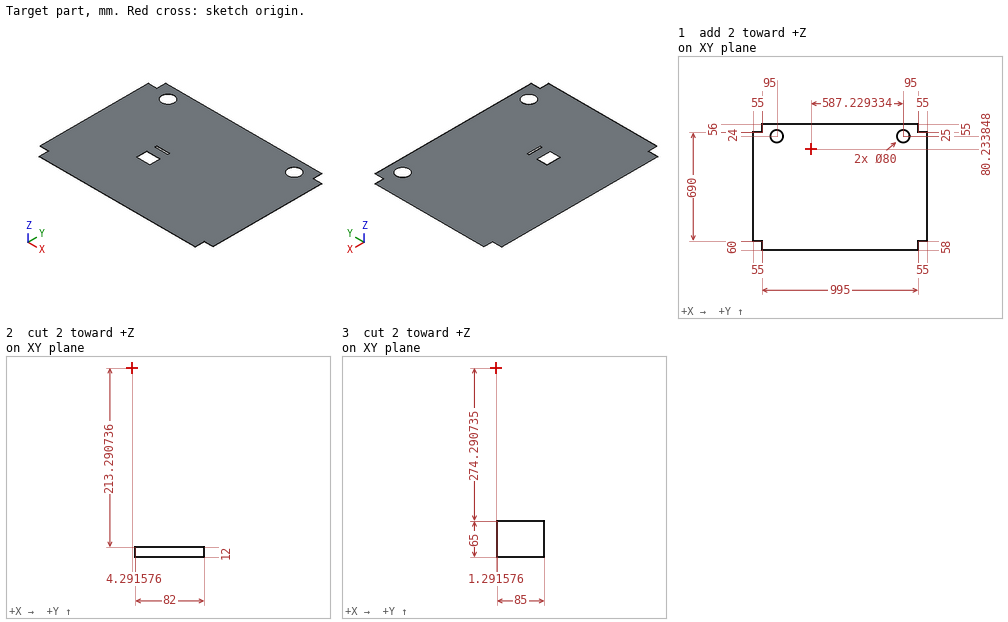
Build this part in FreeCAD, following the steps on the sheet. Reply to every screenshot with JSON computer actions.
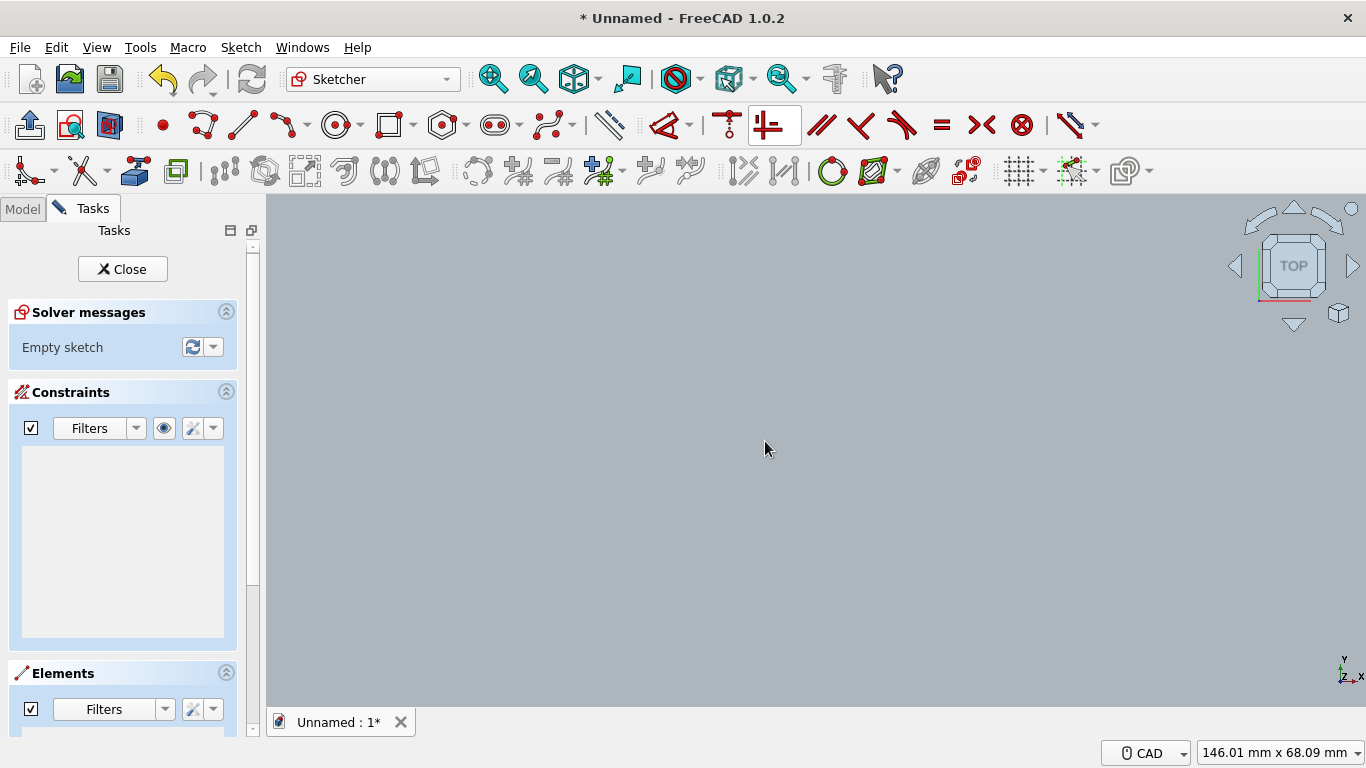
{"action": "left_click", "coordinate": [390, 126]}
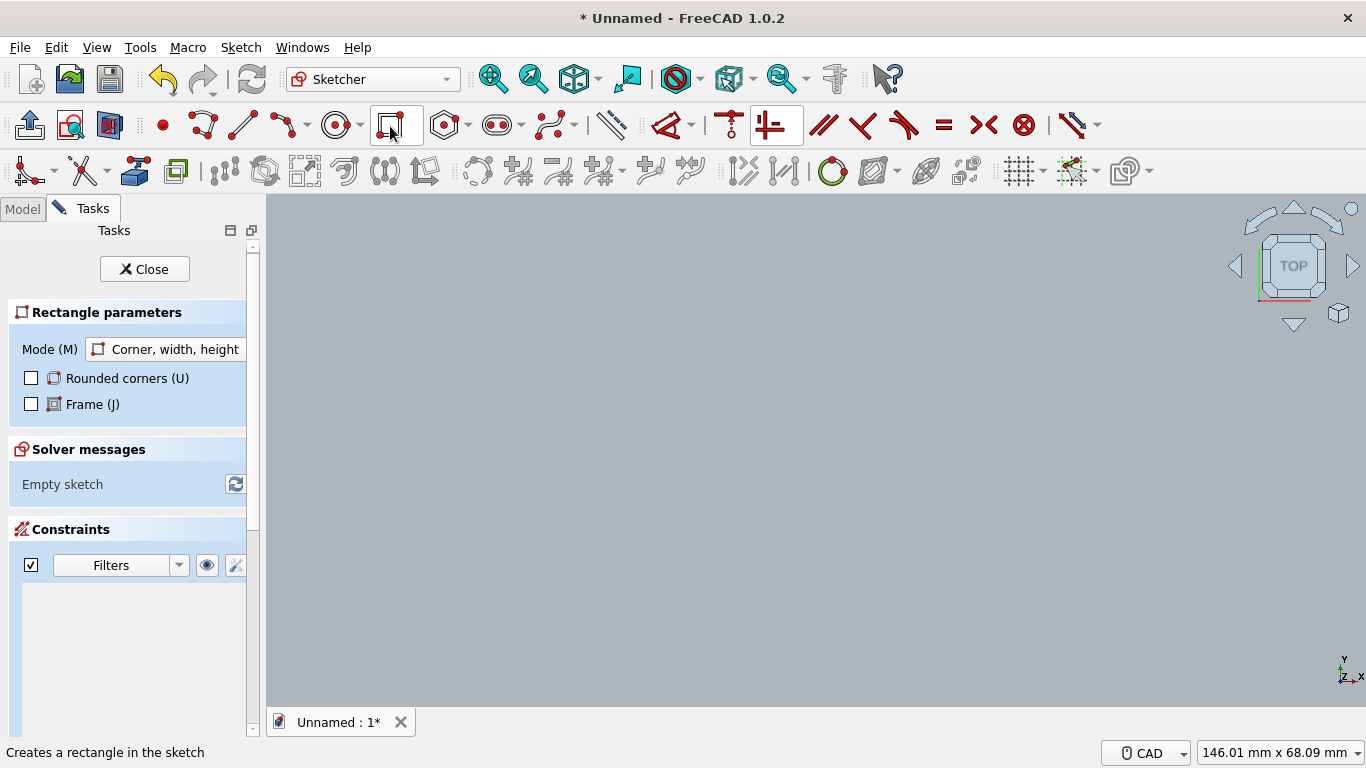
{"action": "left_click", "coordinate": [421, 401]}
{"action": "mouse_move", "coordinate": [1039, 491]}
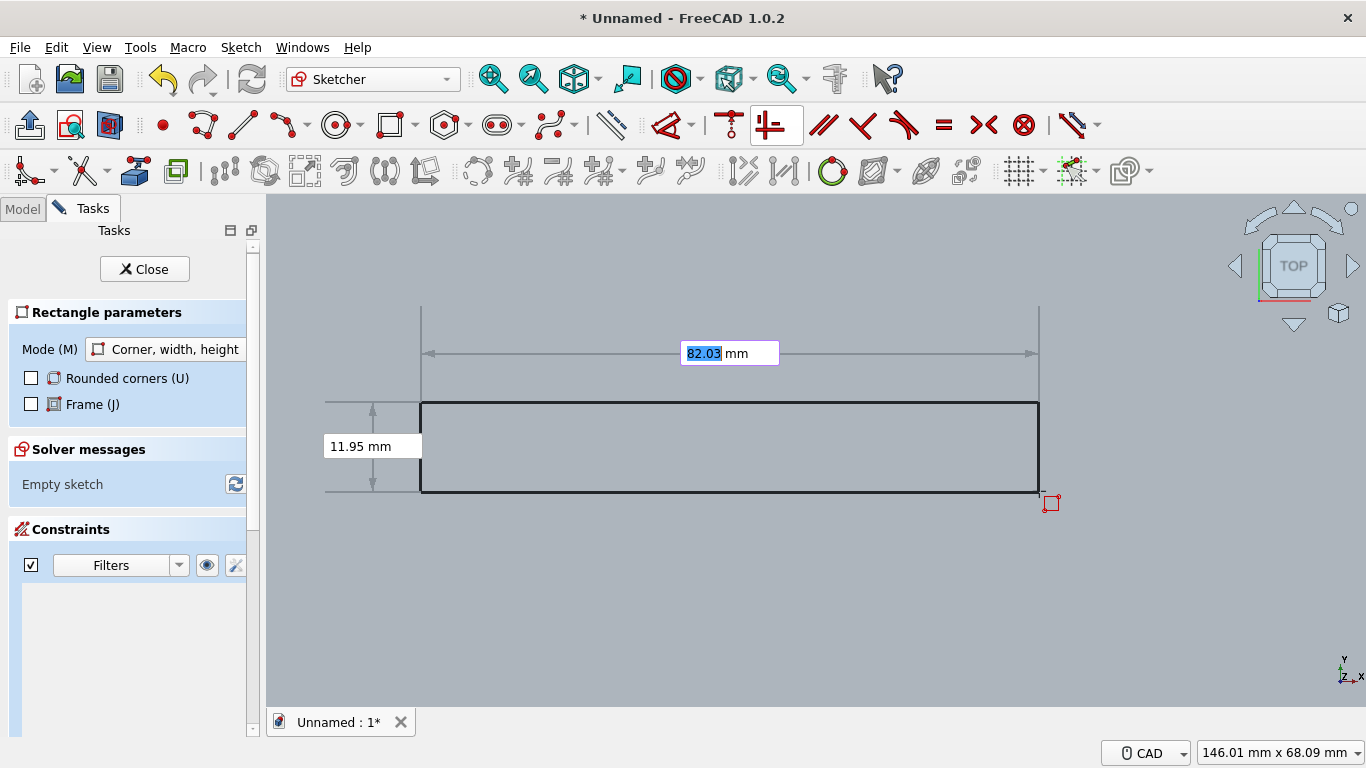
{"action": "type", "text": "82"}
{"action": "key", "text": "Tab"}
{"action": "type", "text": "12"}
{"action": "key", "text": "Return"}
{"action": "key", "text": "Escape"}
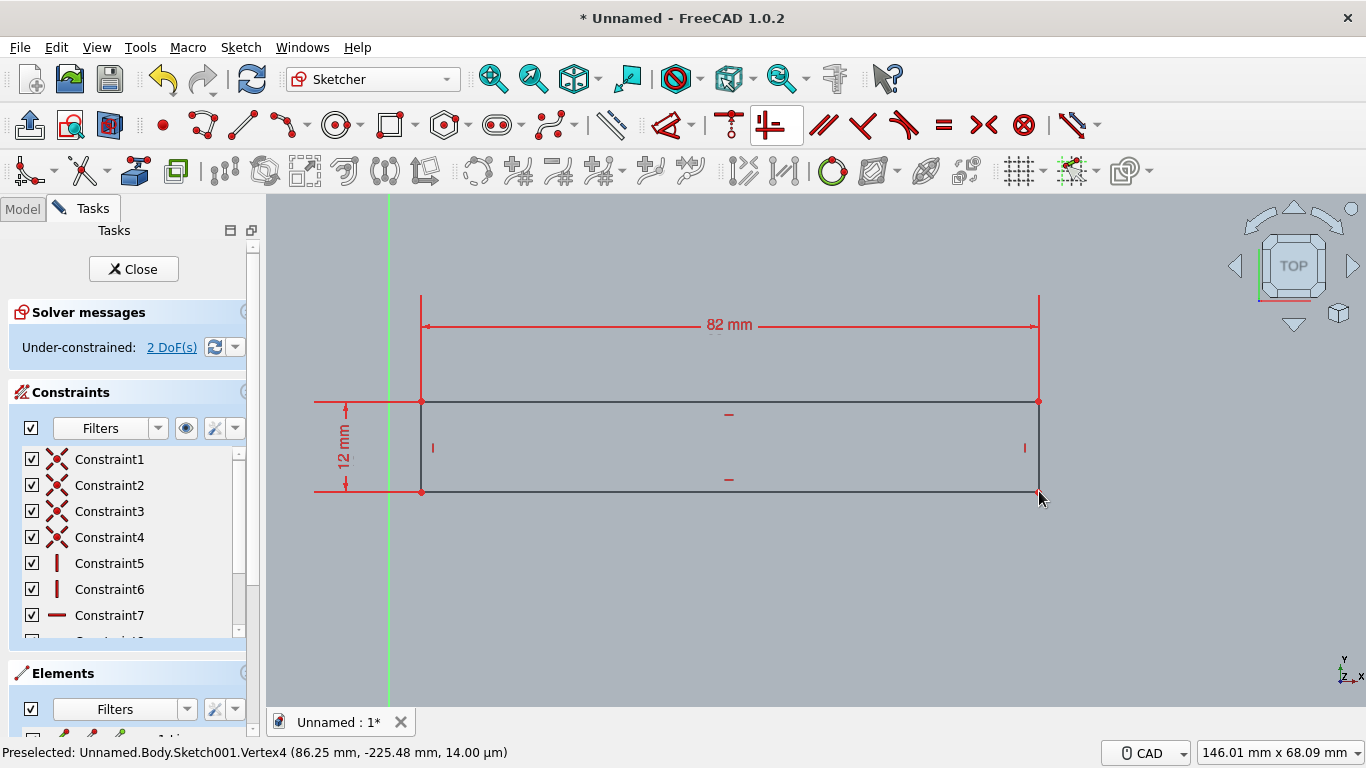
{"action": "left_click", "coordinate": [666, 126]}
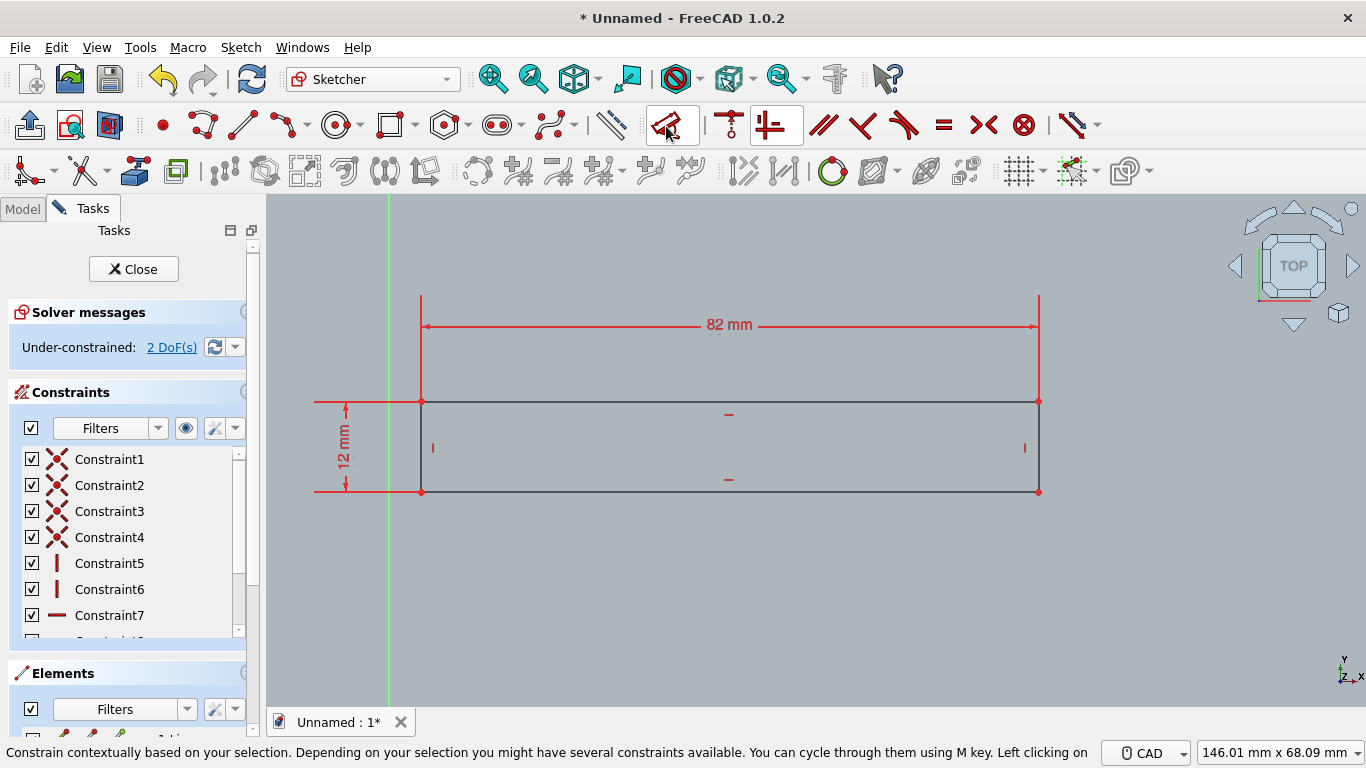
{"action": "scroll", "coordinate": [421, 402], "scroll_direction": "up", "scroll_amount": 2}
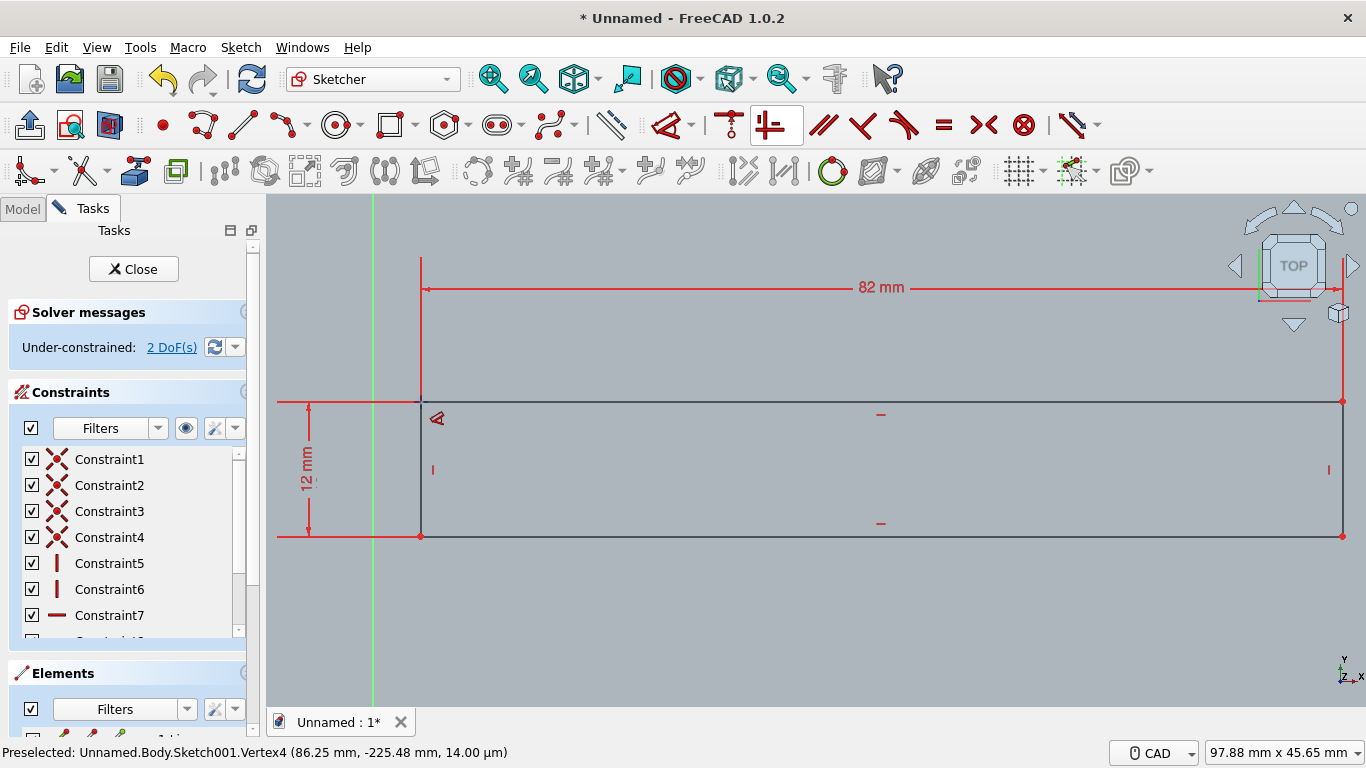
{"action": "left_click", "coordinate": [421, 402]}
{"action": "left_click", "coordinate": [397, 436]}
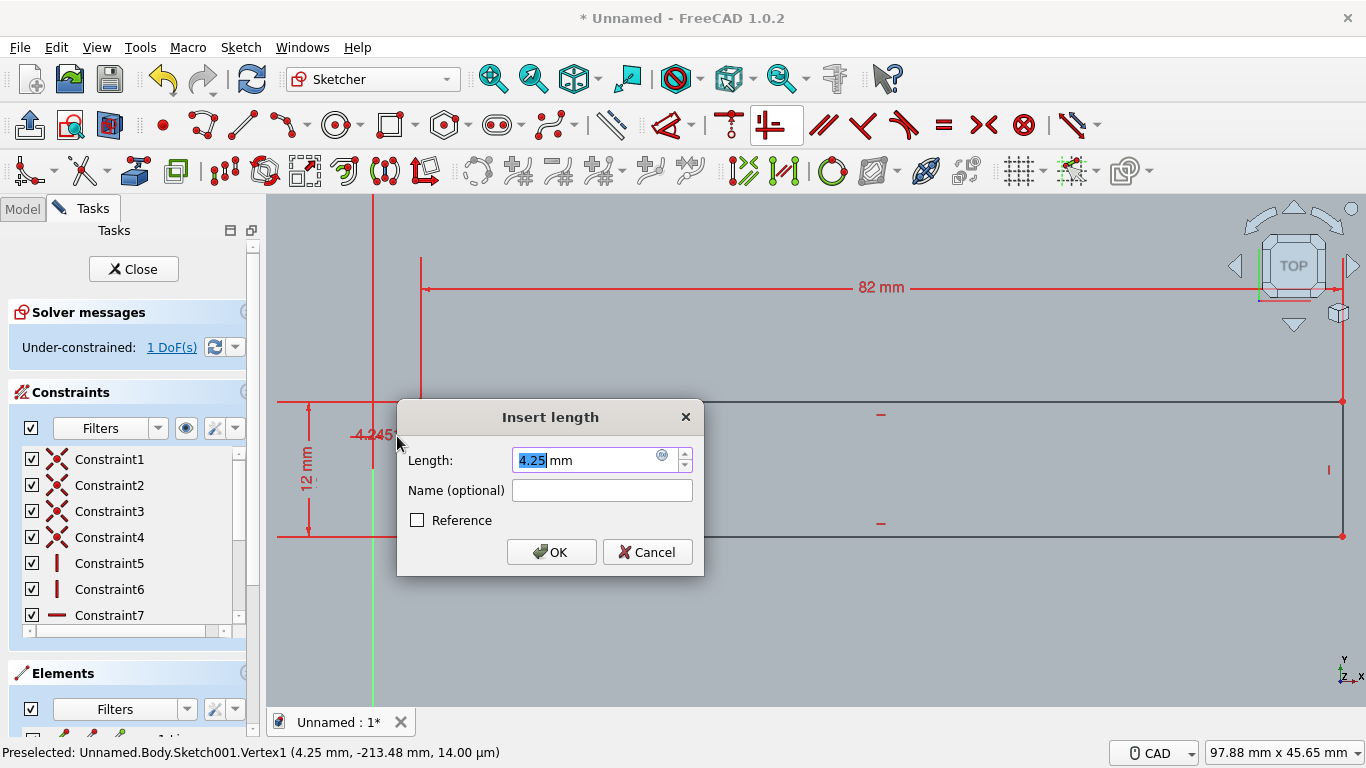
{"action": "type", "text": "4.291576"}
{"action": "key", "text": "Return"}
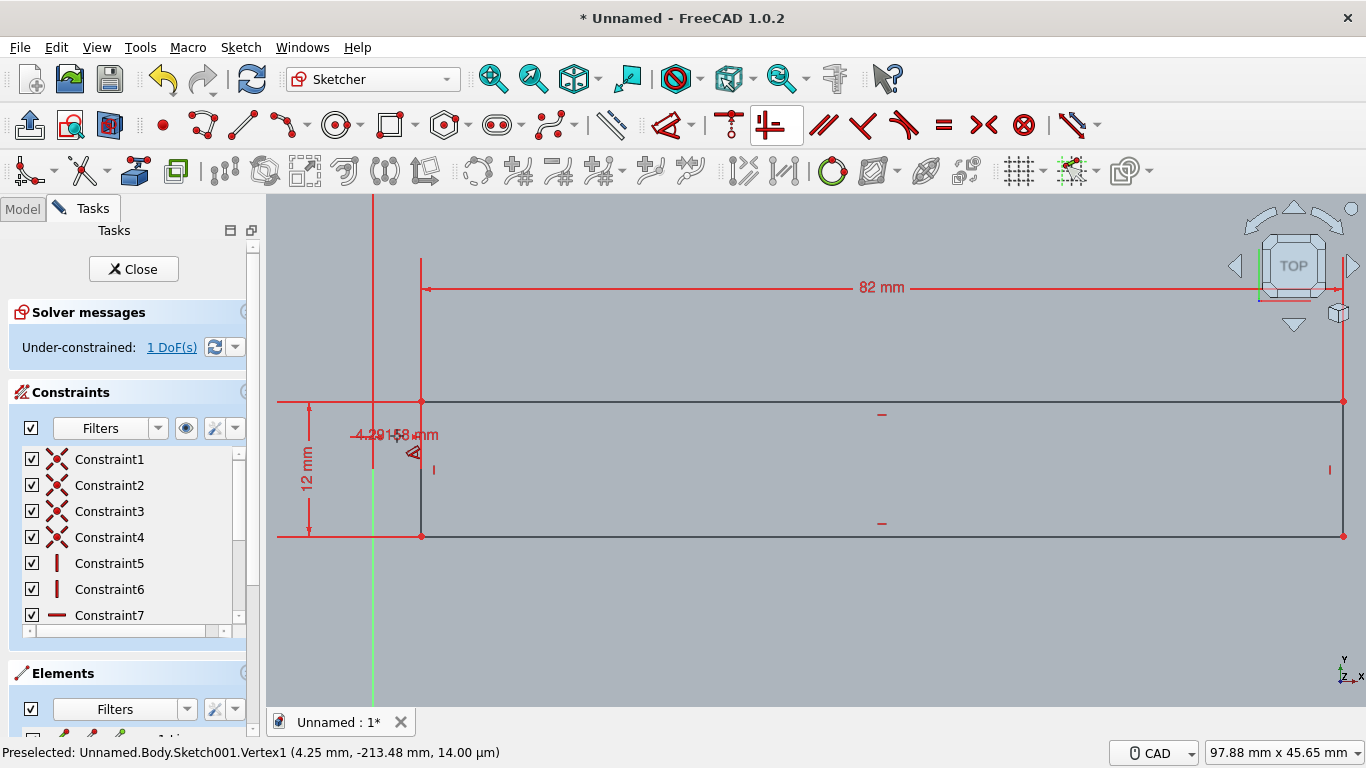
{"action": "left_click", "coordinate": [421, 402]}
{"action": "left_click", "coordinate": [339, 312]}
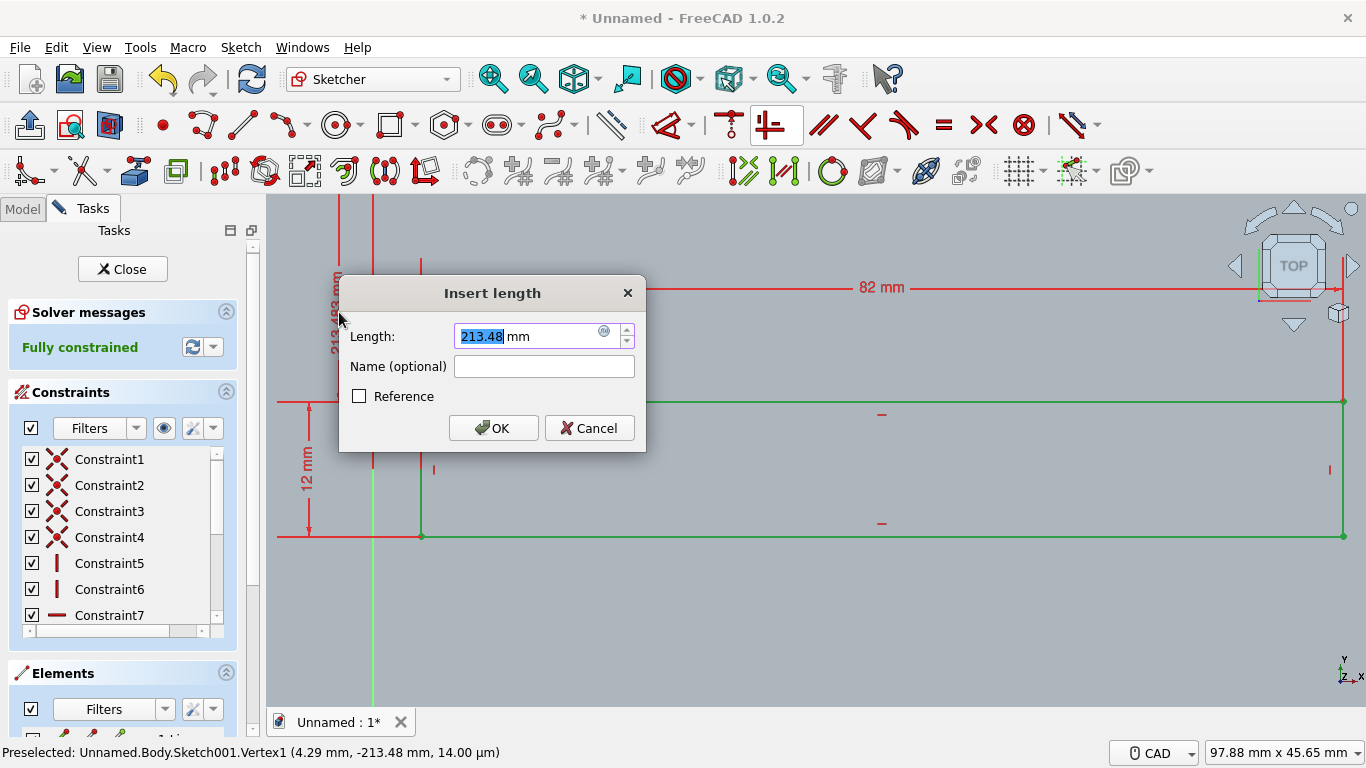
{"action": "type", "text": "213.290736"}
{"action": "key", "text": "Return"}
{"action": "key", "text": "Escape"}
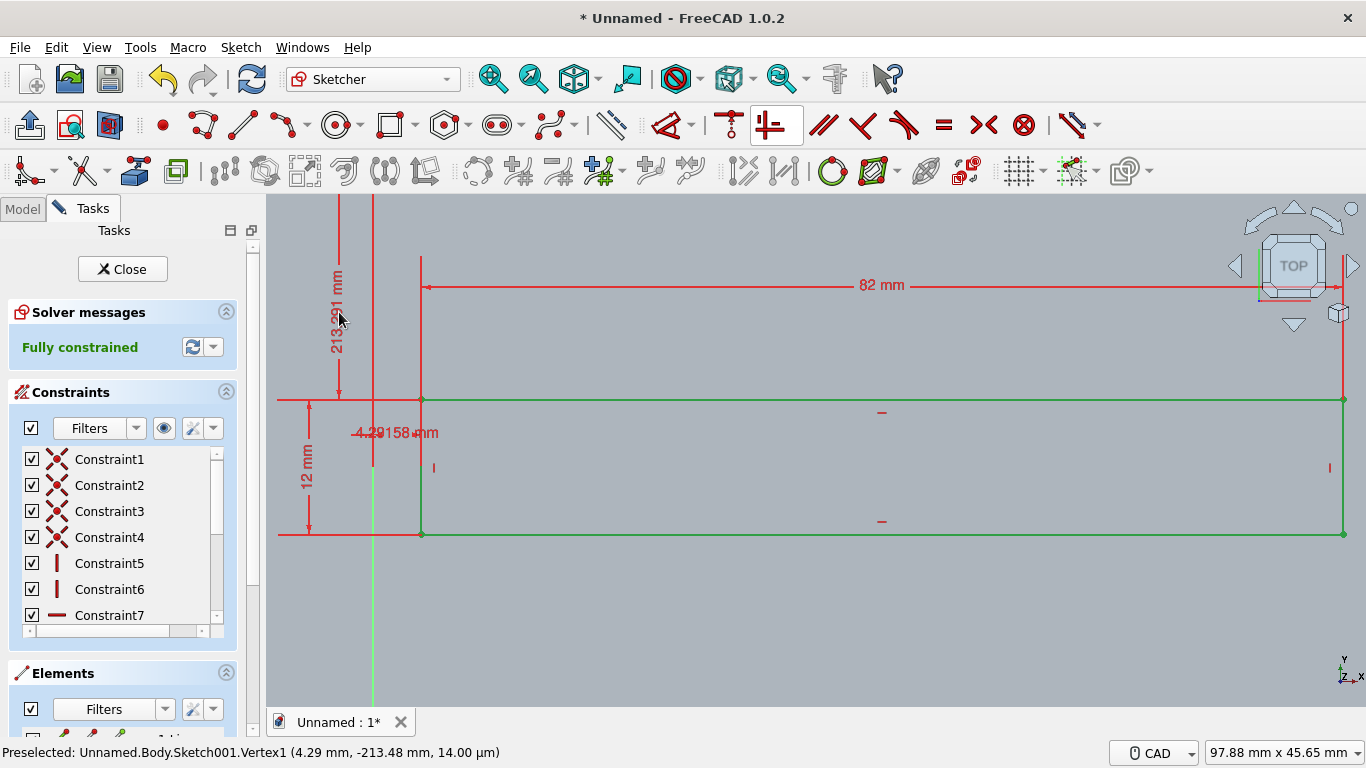
{"action": "left_click", "coordinate": [123, 269]}